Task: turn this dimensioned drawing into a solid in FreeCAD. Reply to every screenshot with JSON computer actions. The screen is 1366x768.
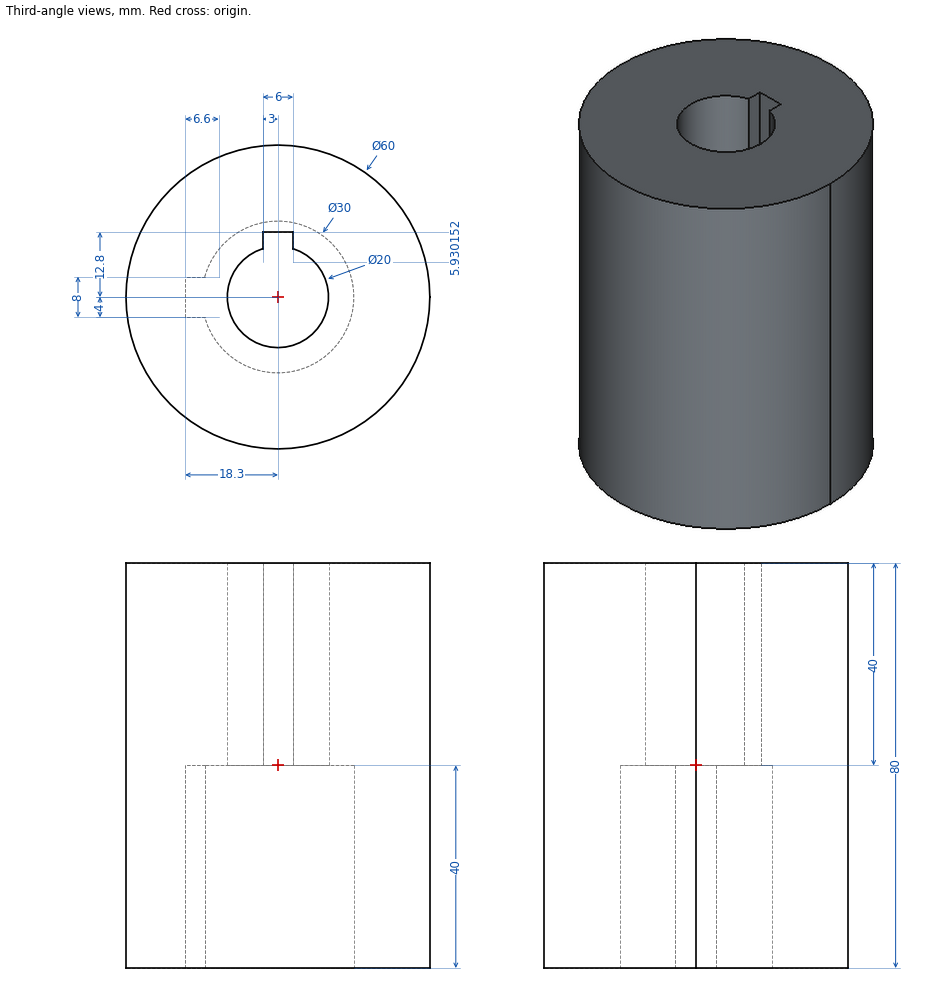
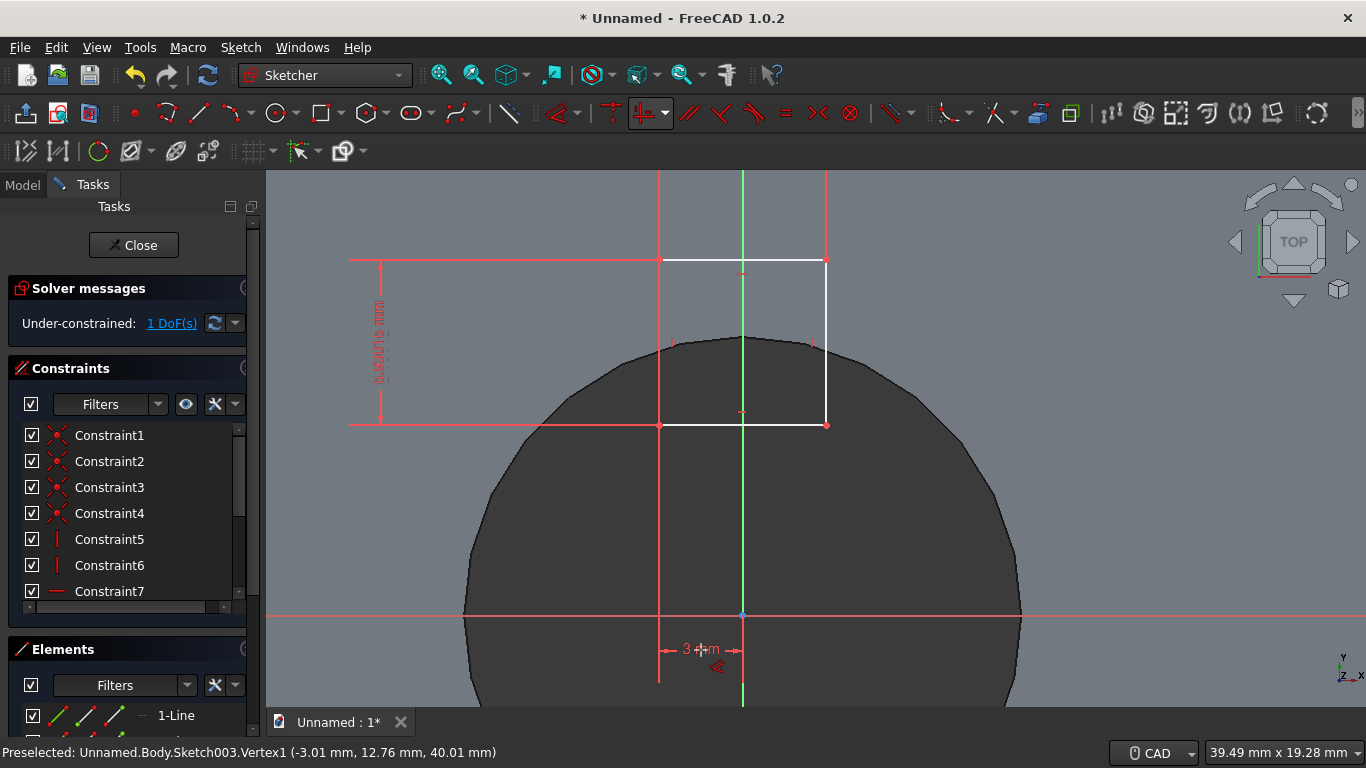
{"action": "left_click", "coordinate": [659, 260]}
{"action": "left_click", "coordinate": [625, 438]}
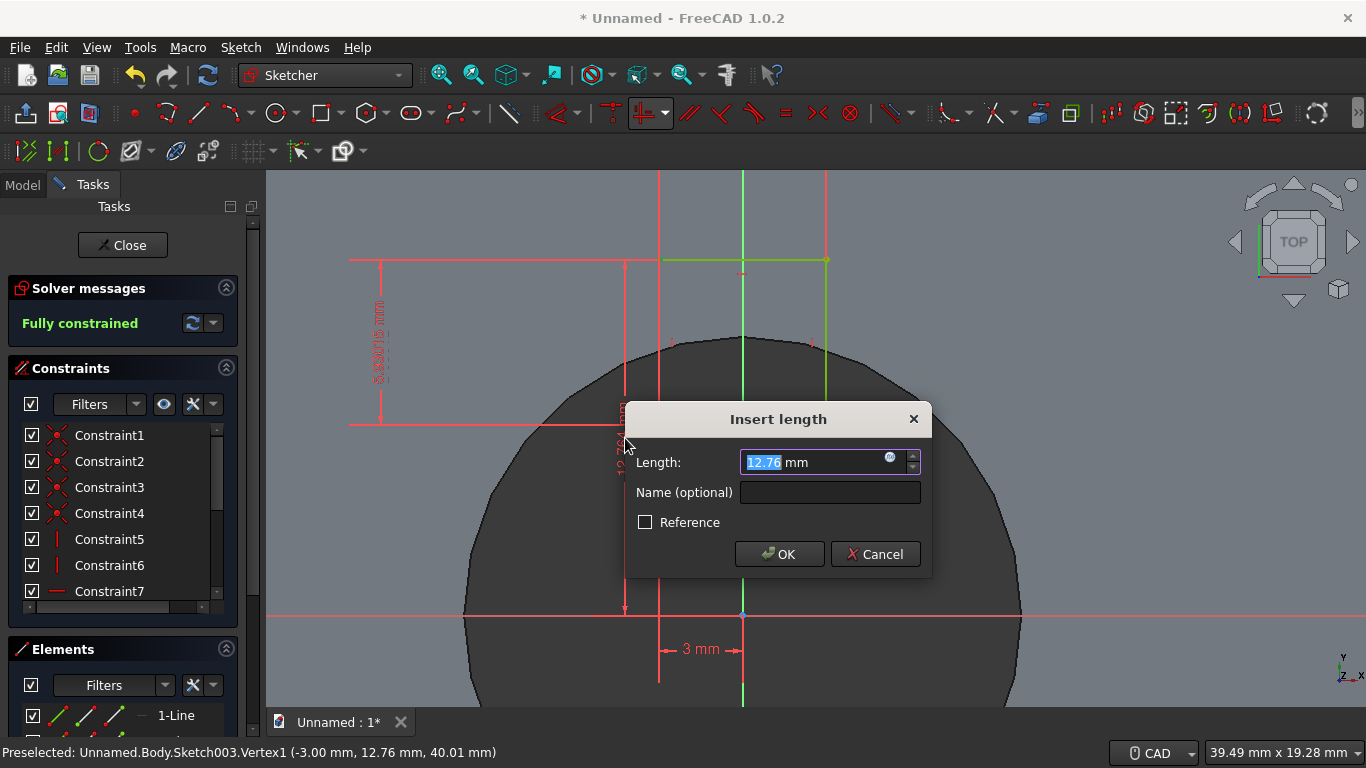
{"action": "type", "text": "12.8"}
{"action": "key", "text": "Return"}
{"action": "key", "text": "Escape"}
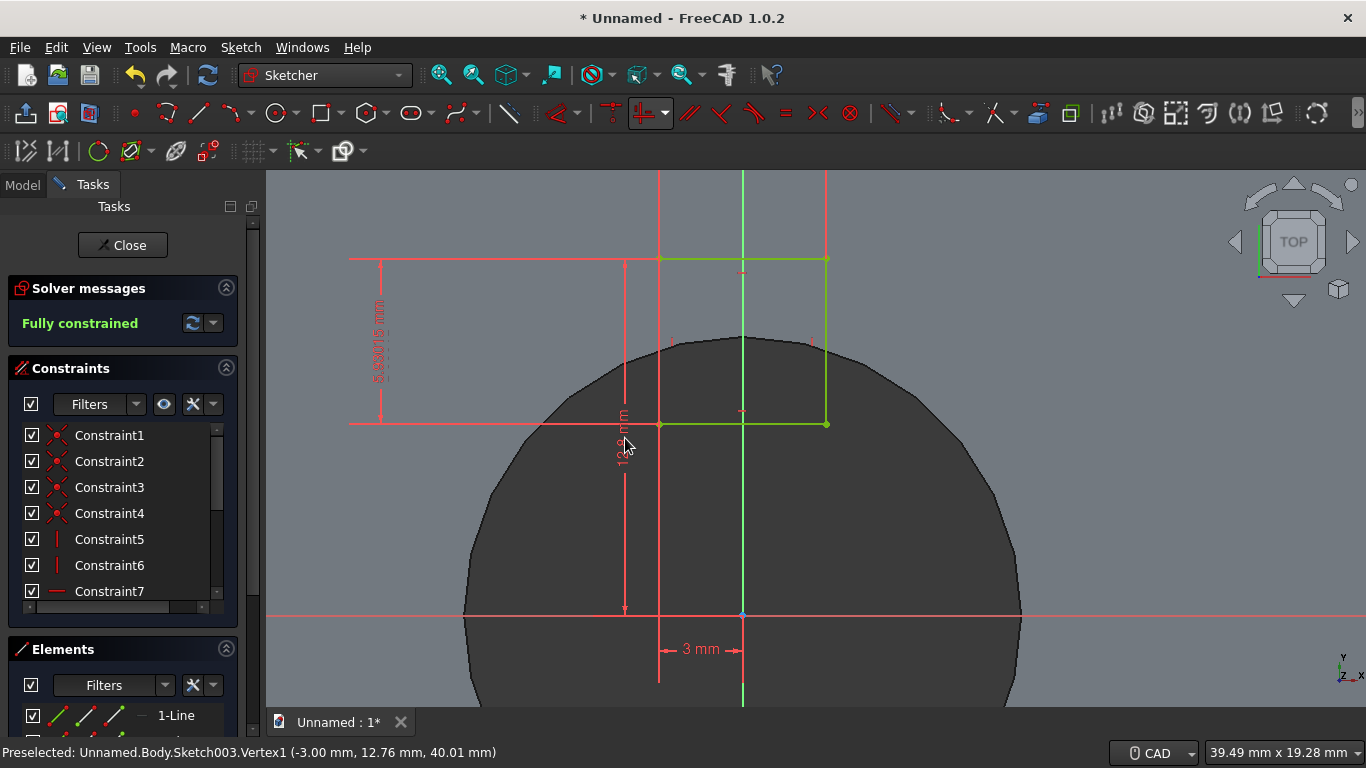
{"action": "left_click", "coordinate": [123, 245]}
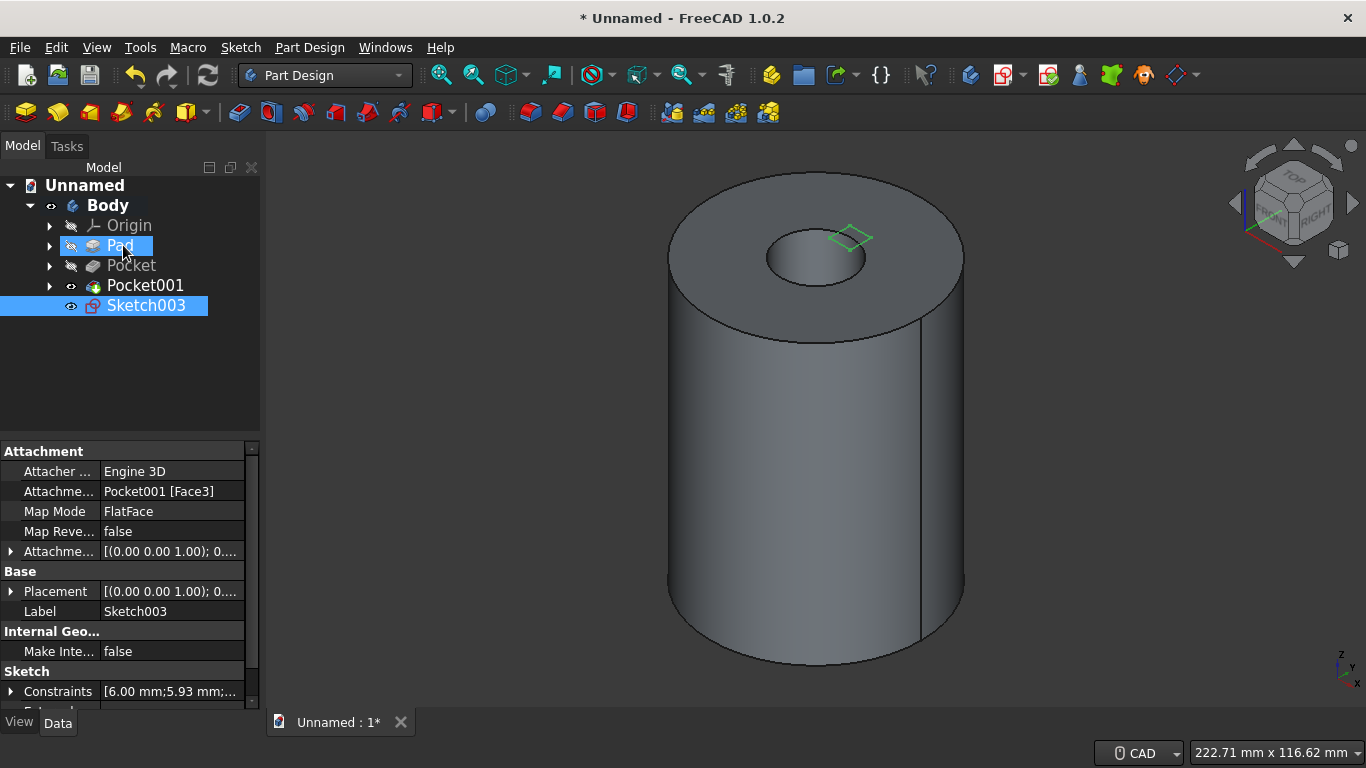
{"action": "left_click", "coordinate": [240, 112]}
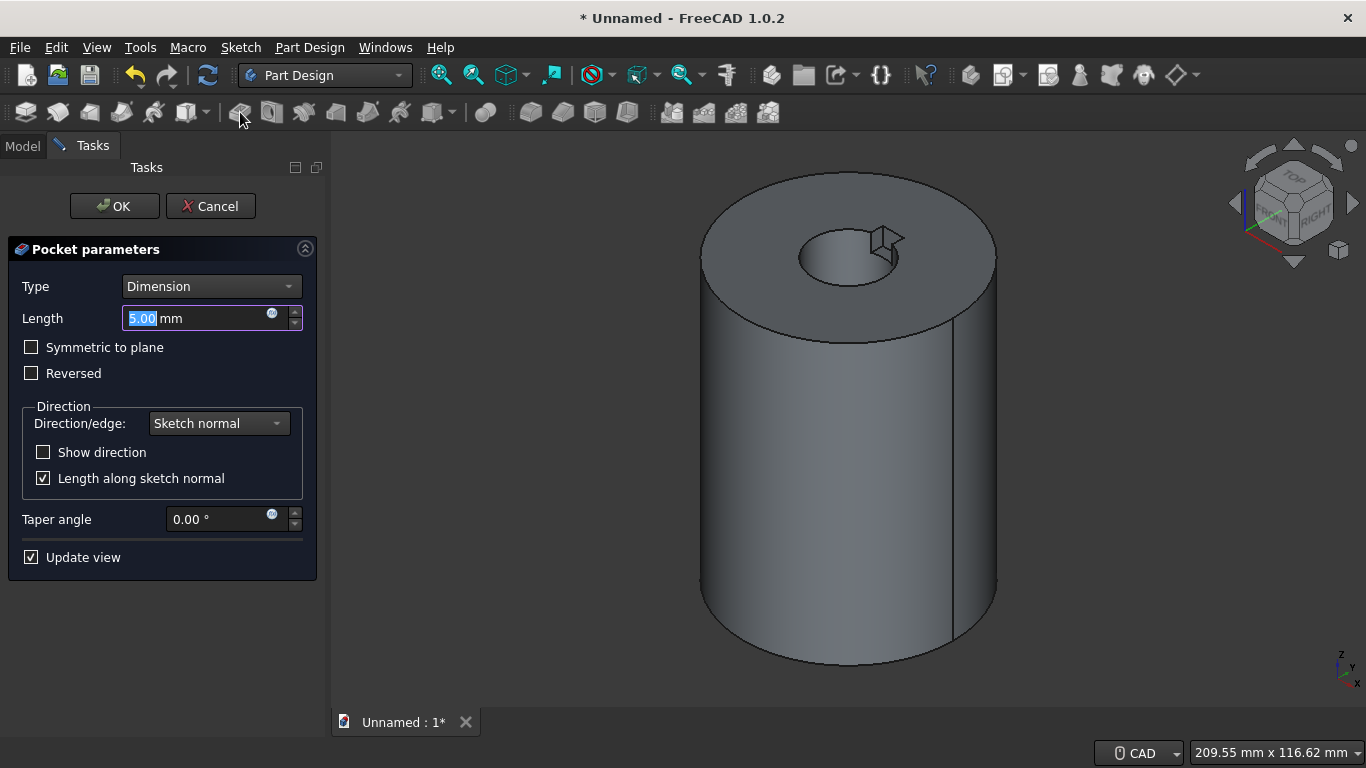
{"action": "type", "text": "40"}
{"action": "key", "text": "Tab"}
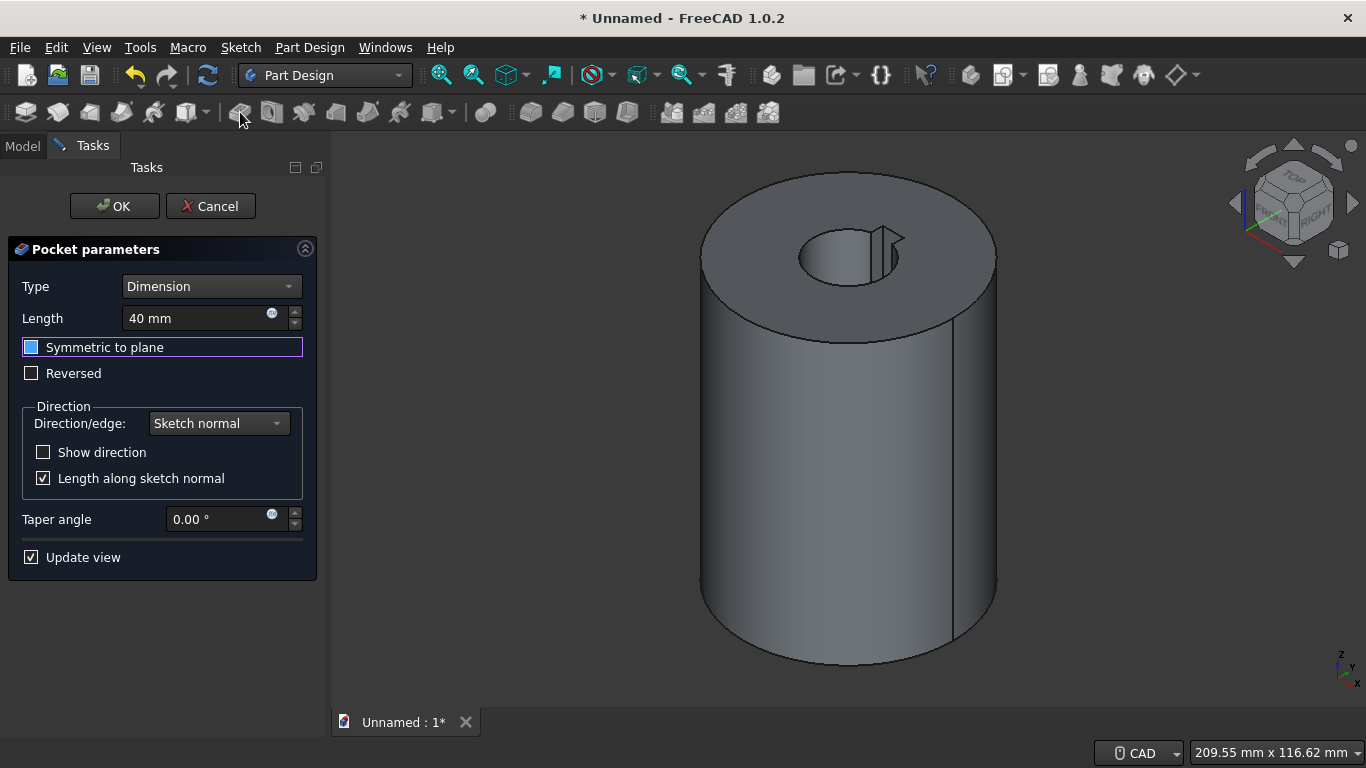
{"action": "left_click", "coordinate": [115, 206]}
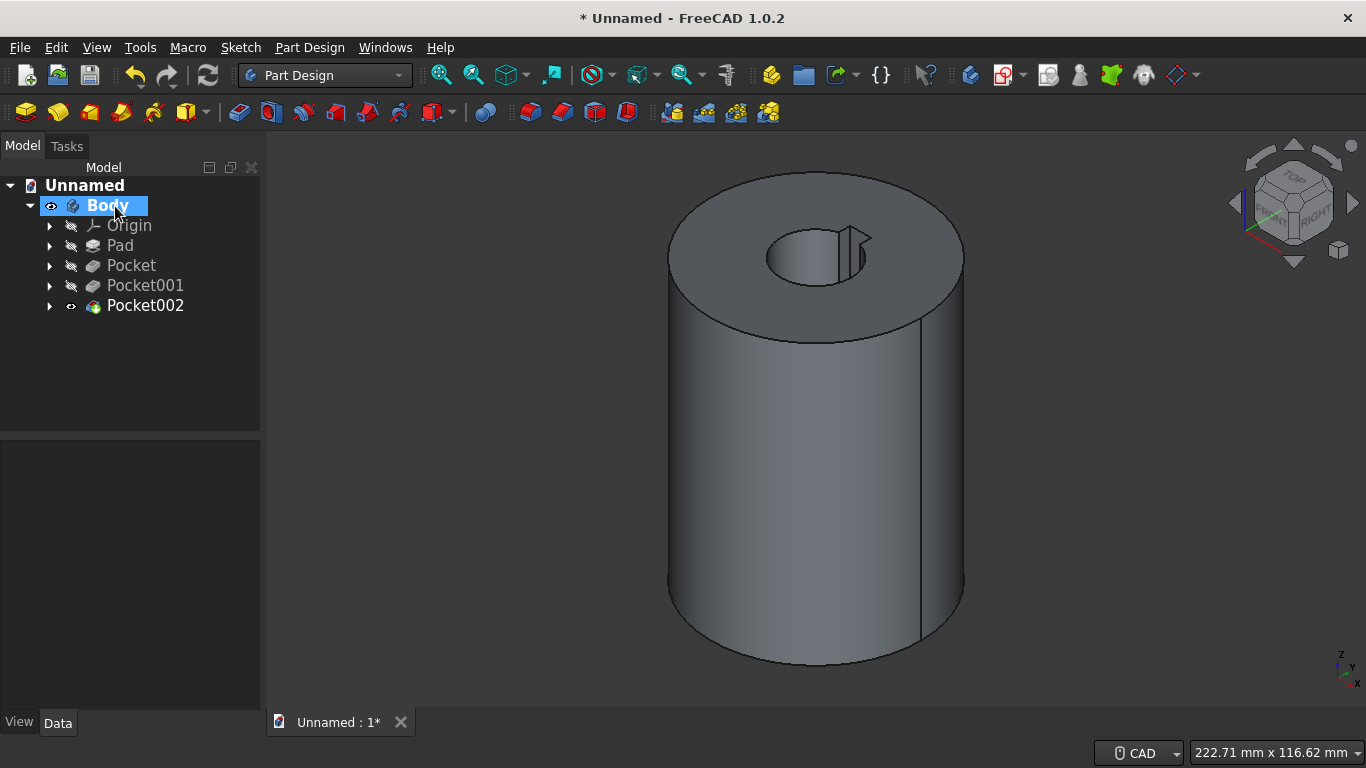
{"action": "key", "text": "5"}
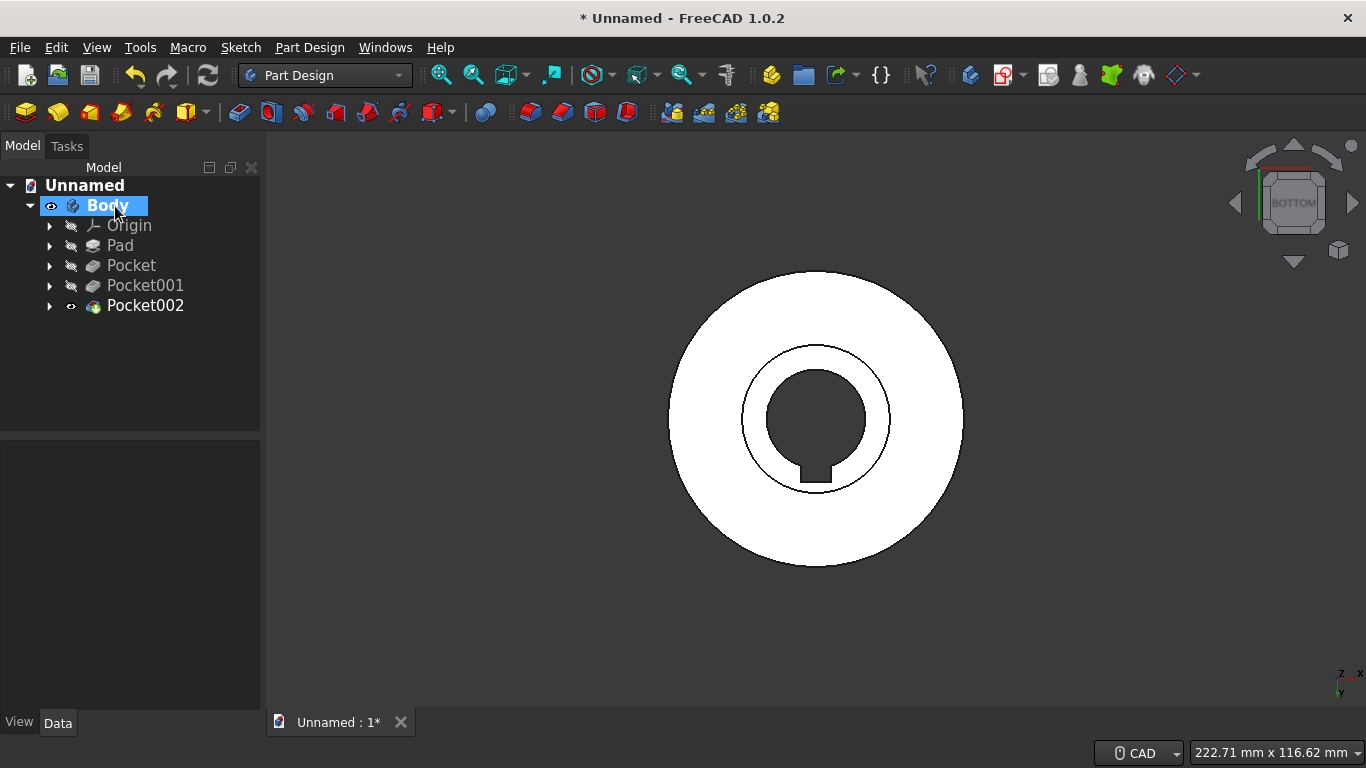
{"action": "left_click", "coordinate": [731, 333]}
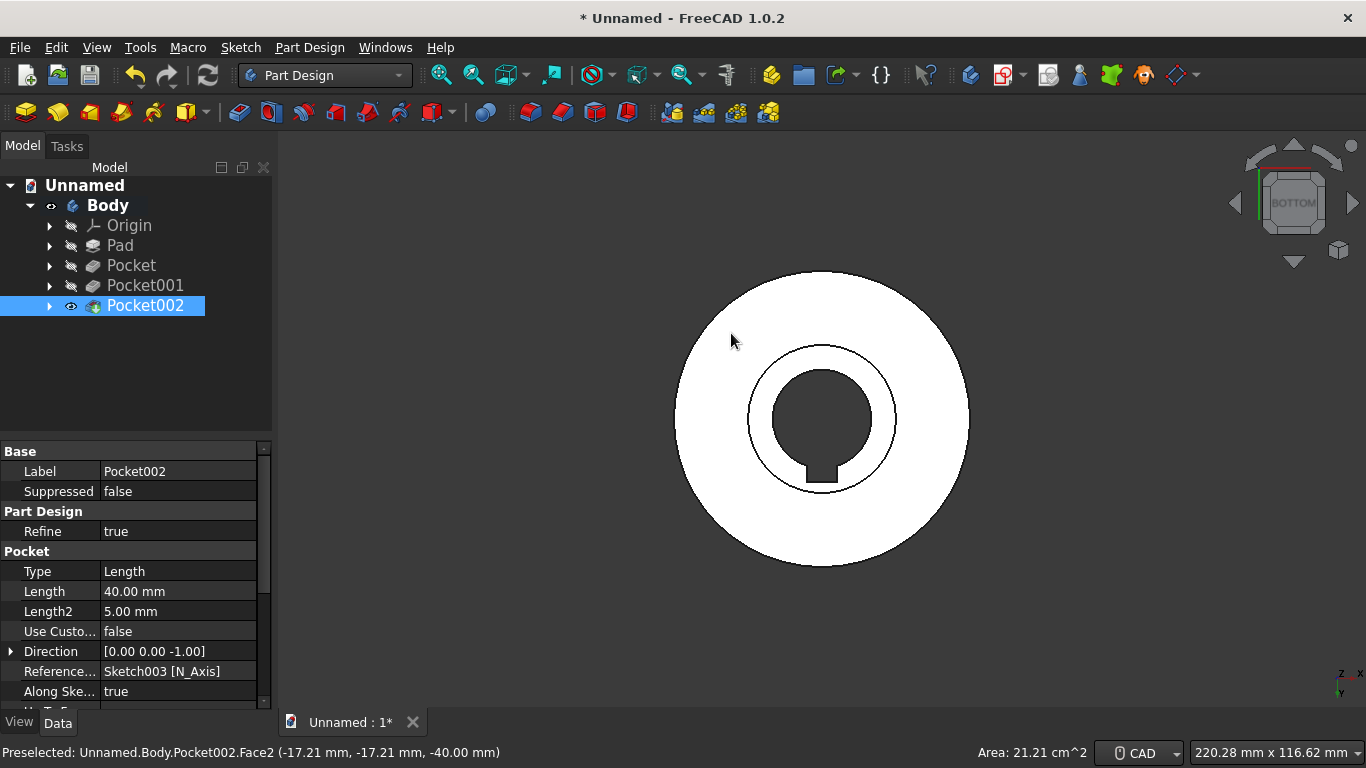
{"action": "left_click", "coordinate": [1004, 76]}